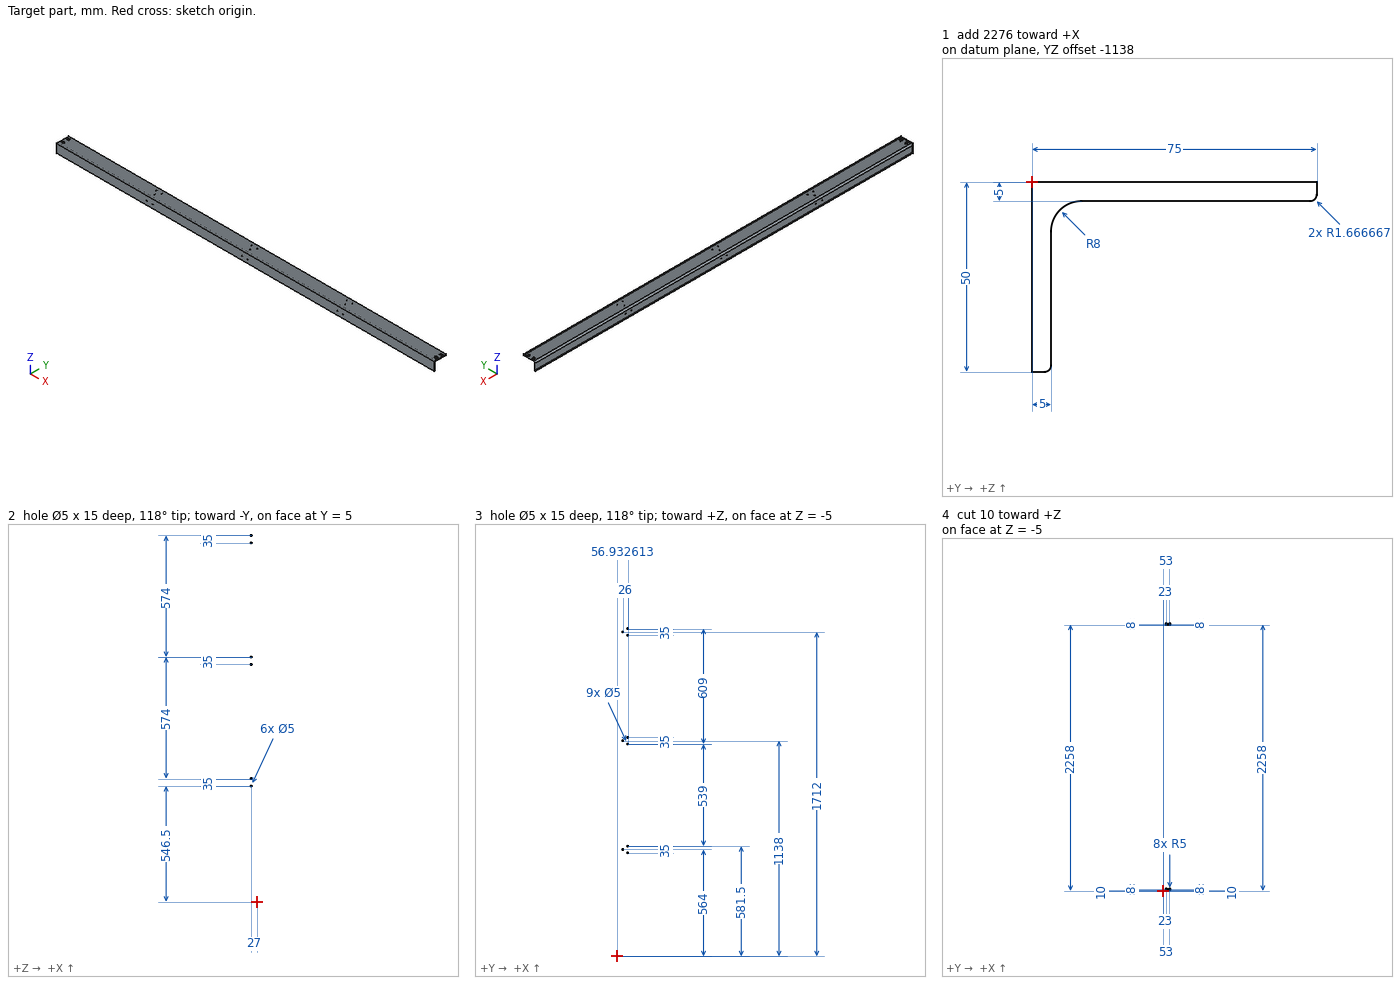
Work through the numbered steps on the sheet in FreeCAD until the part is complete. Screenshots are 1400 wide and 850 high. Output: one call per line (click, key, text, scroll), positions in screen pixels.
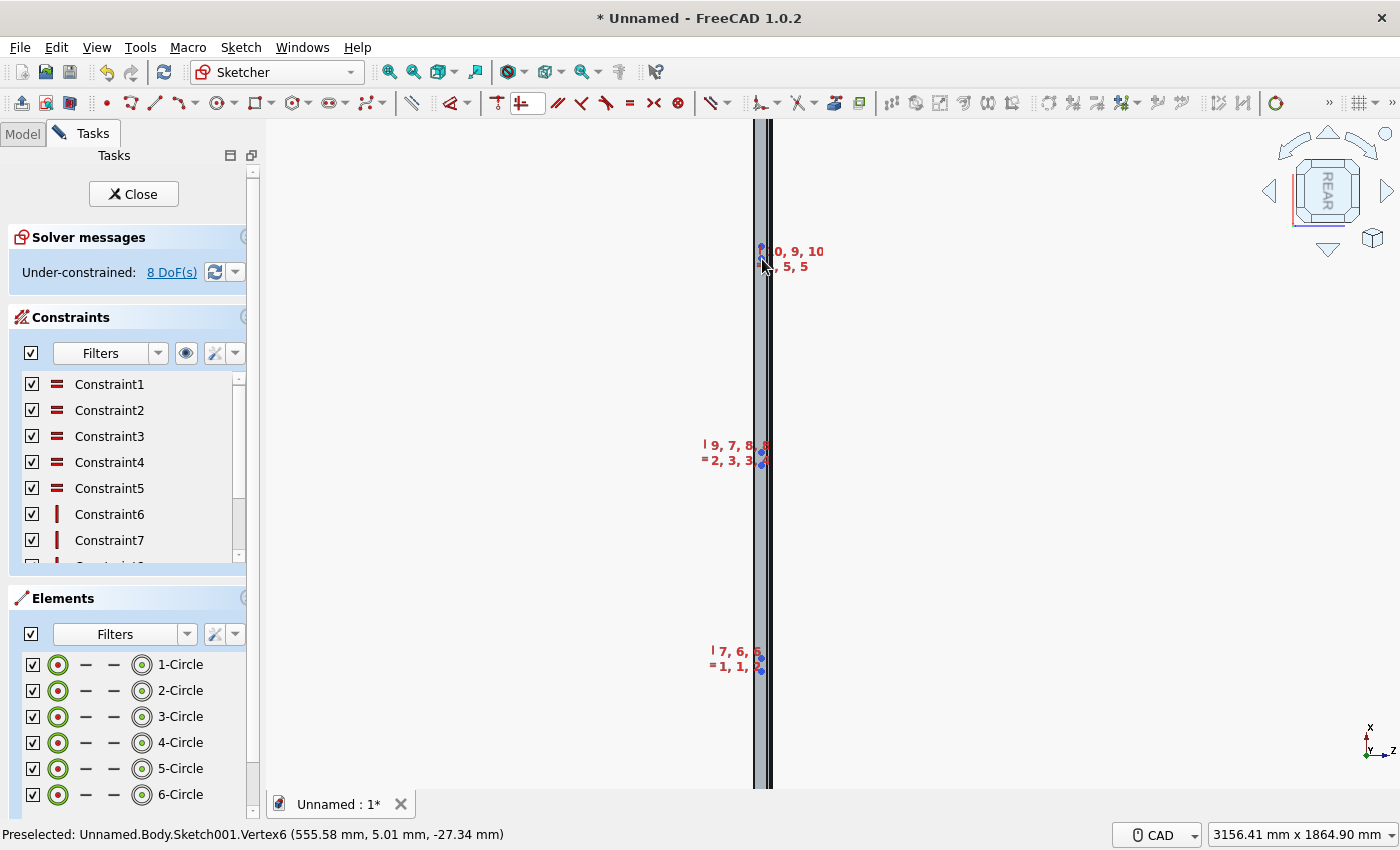
click(450, 104)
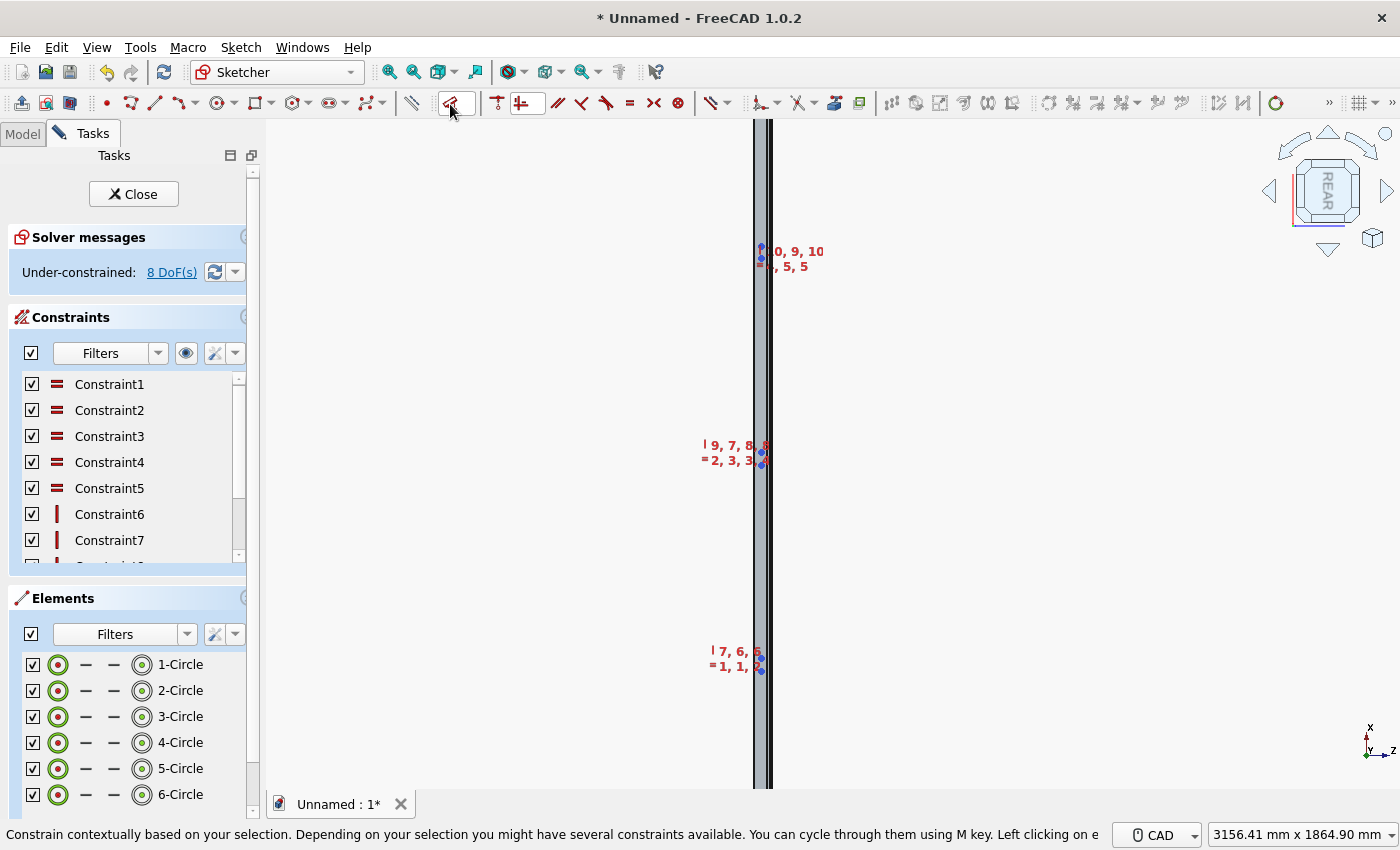
scroll(763, 670, up, 16)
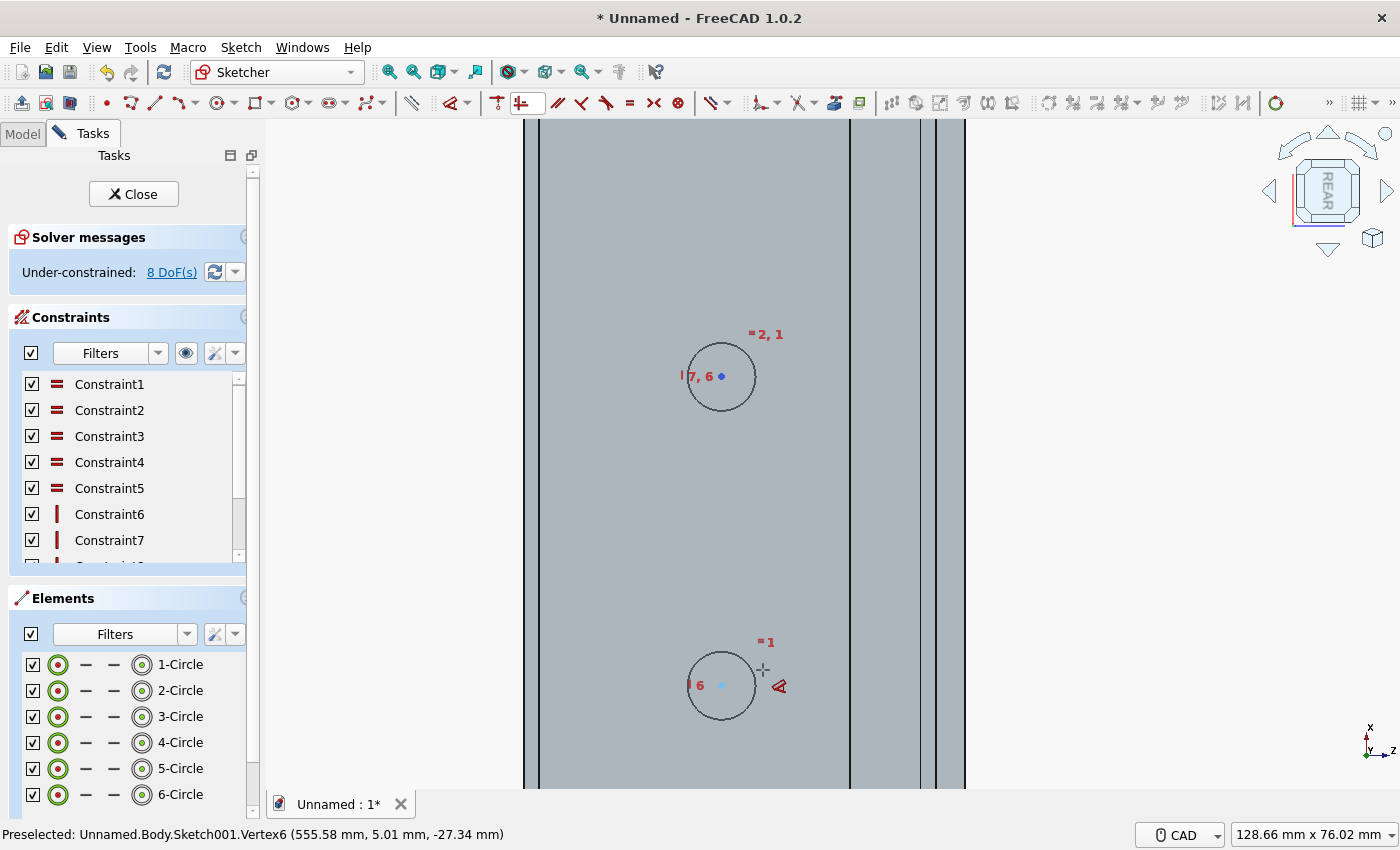
click(746, 662)
click(769, 640)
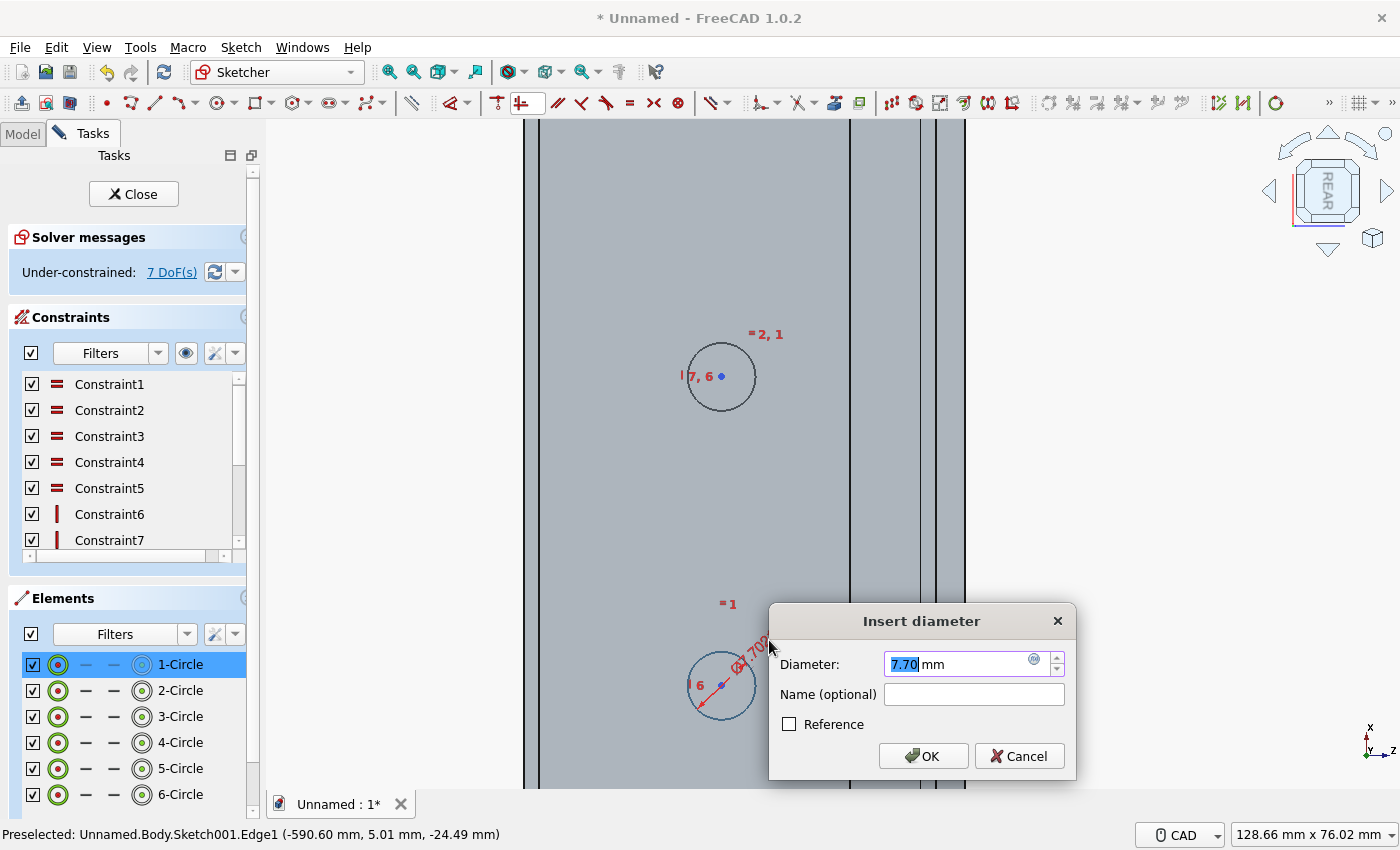
text(5)
key(Return)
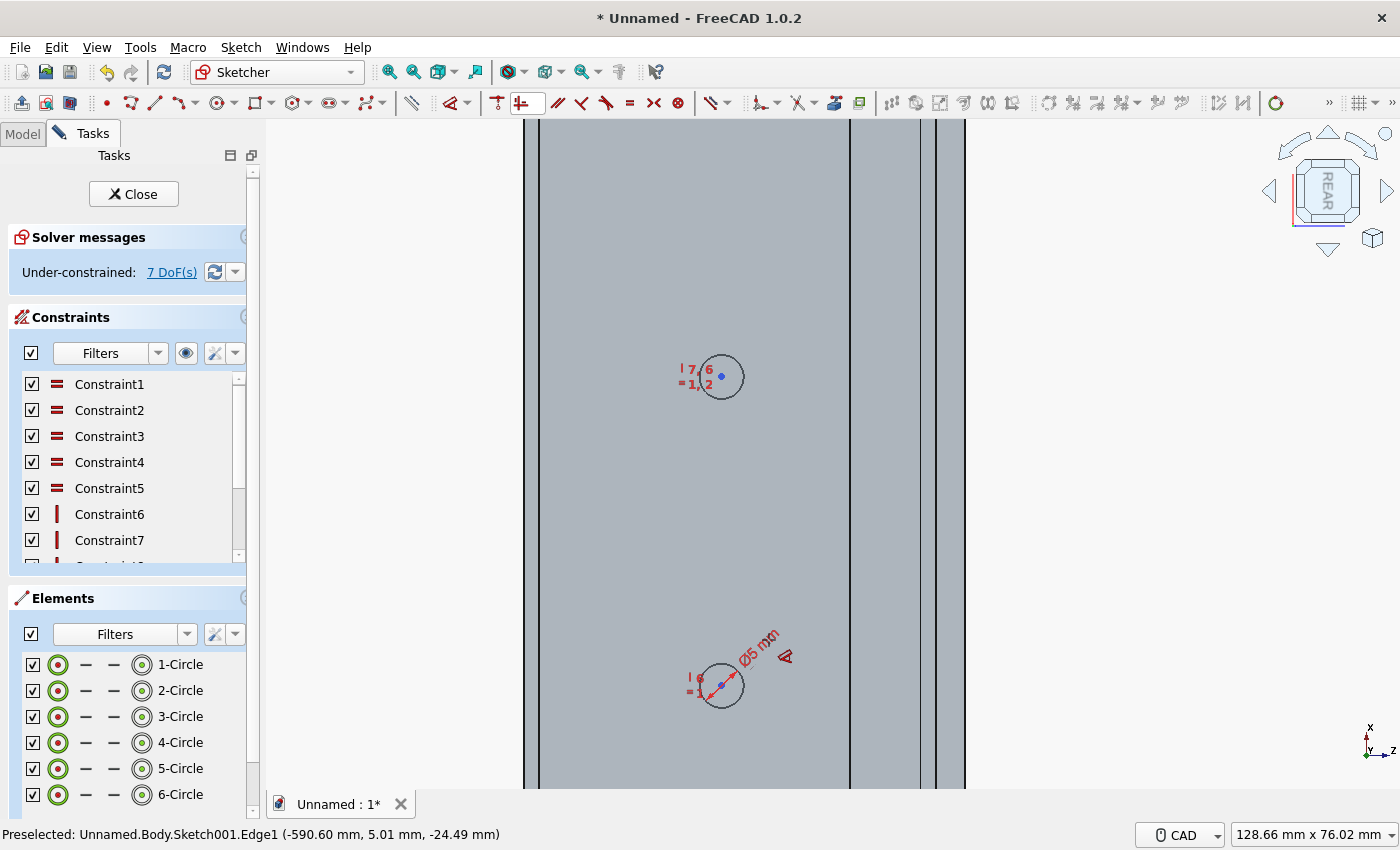
scroll(762, 544, down, 17)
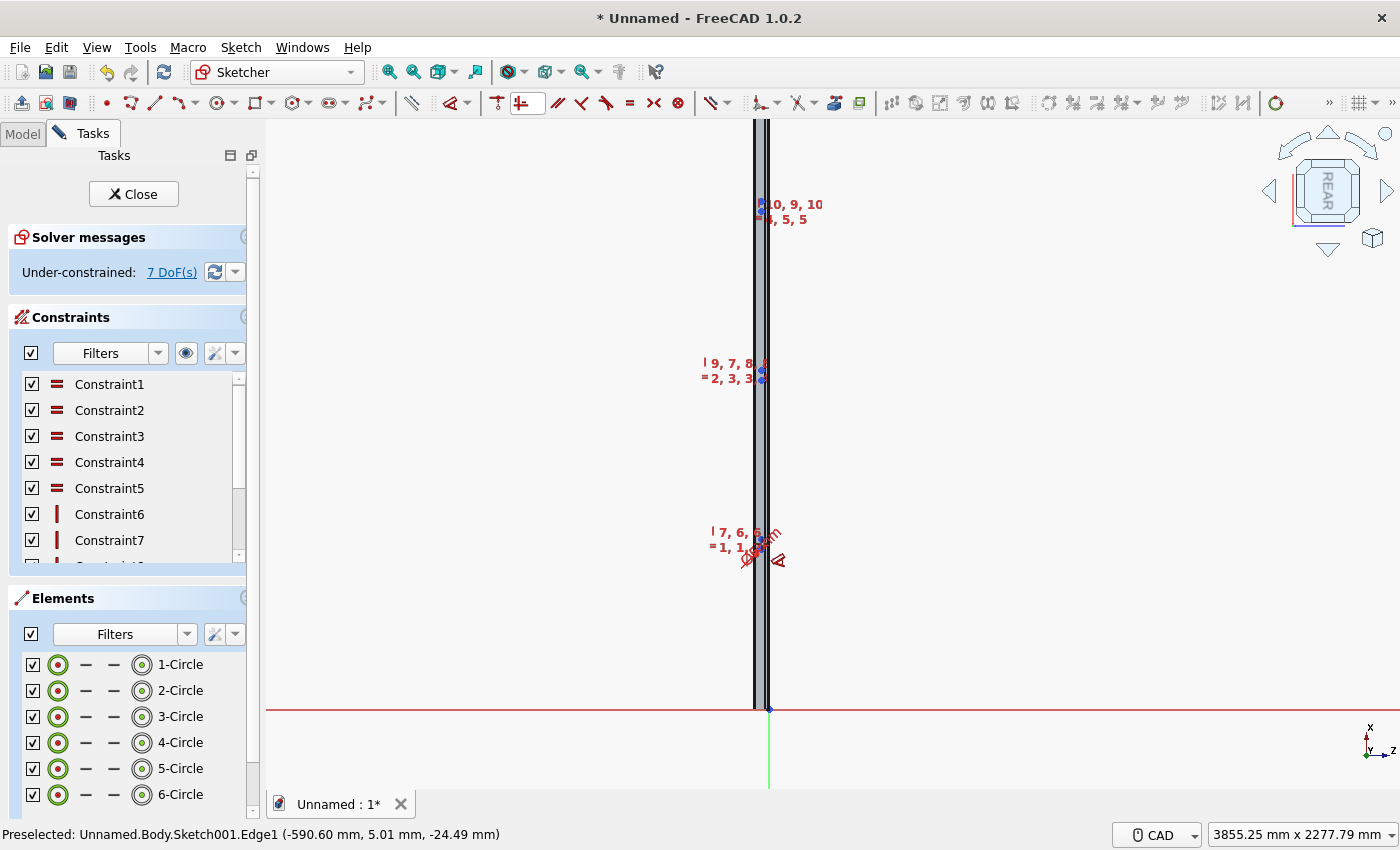
scroll(761, 549, up, 9)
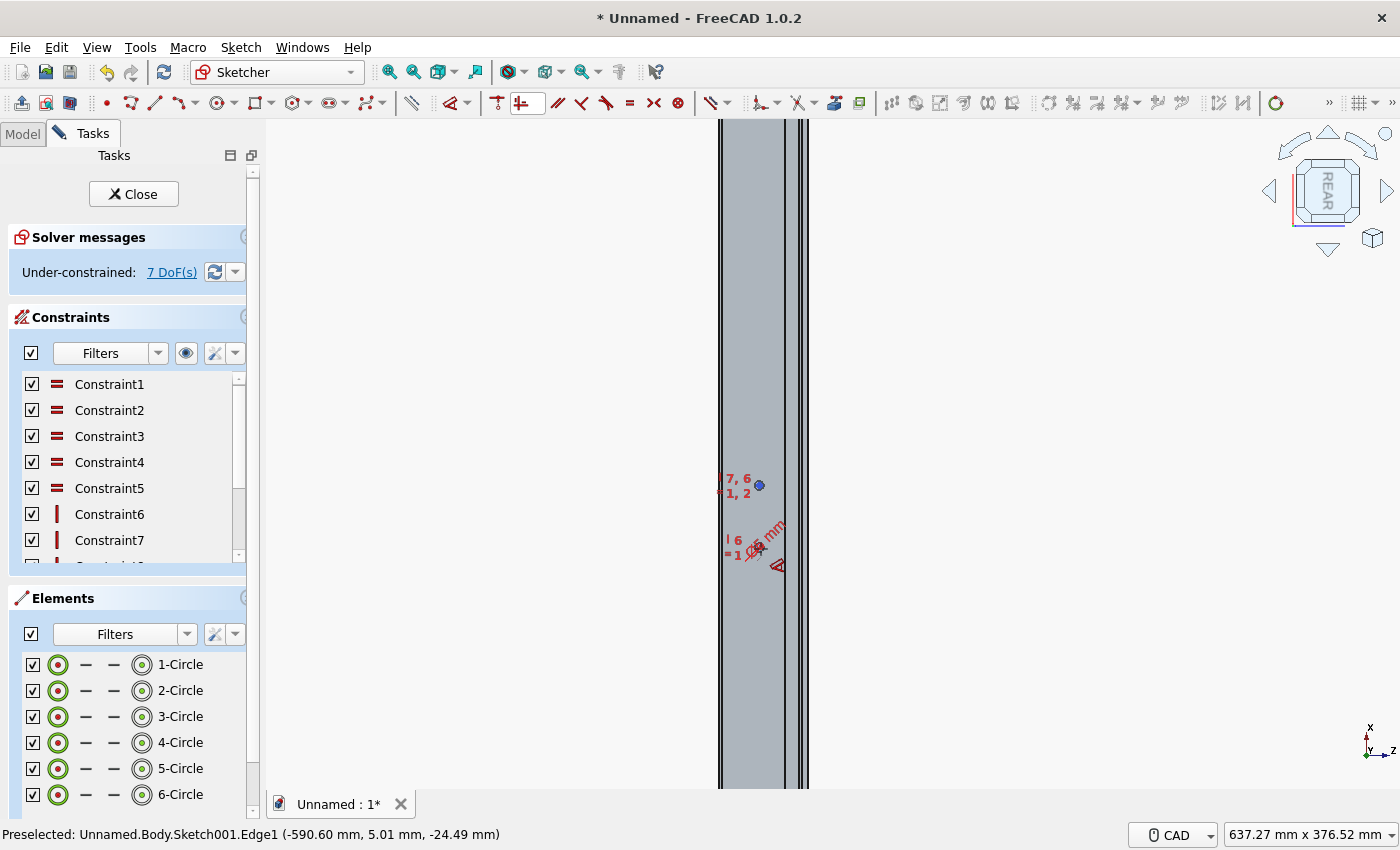
click(759, 548)
click(784, 514)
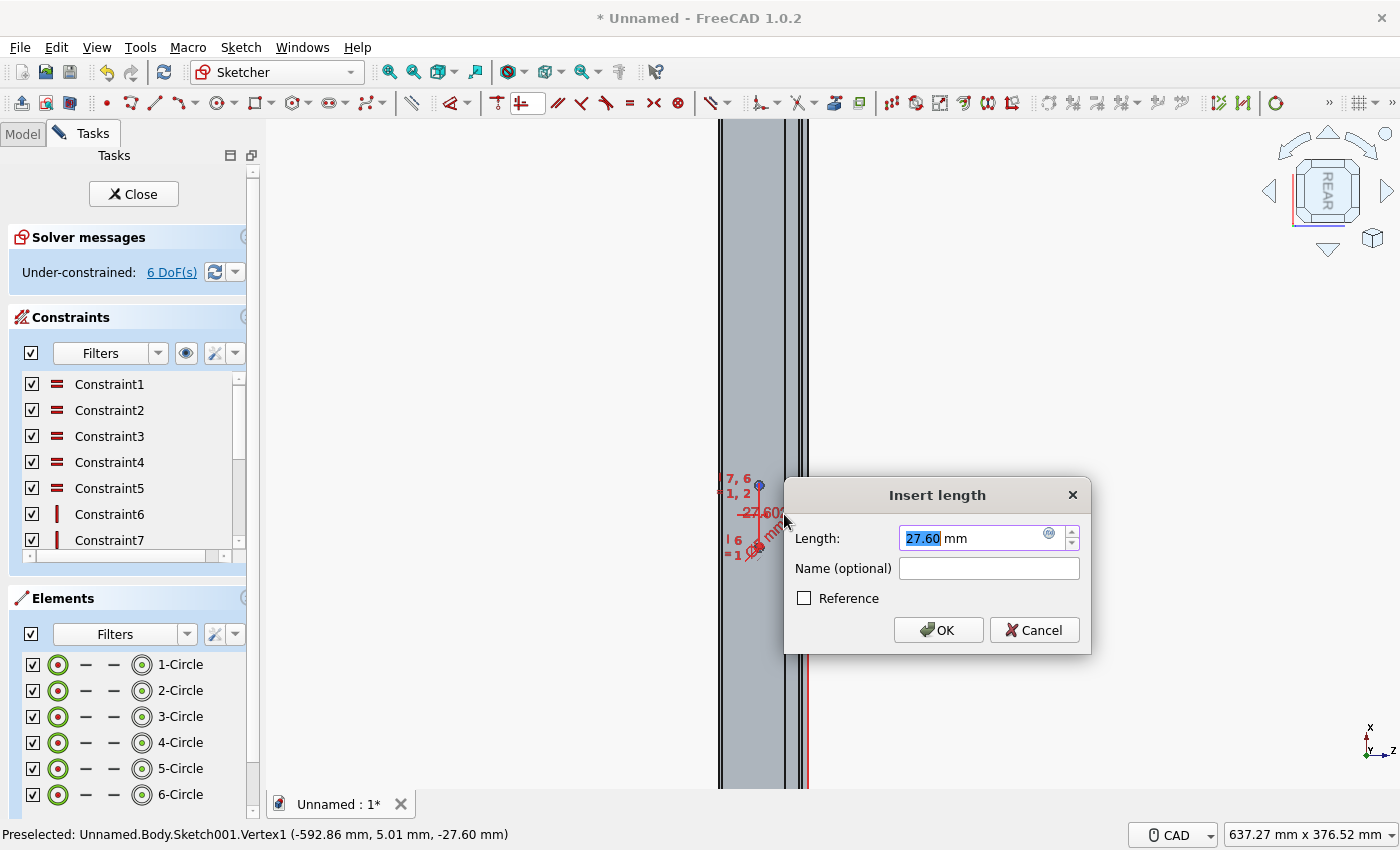
text(27)
key(Return)